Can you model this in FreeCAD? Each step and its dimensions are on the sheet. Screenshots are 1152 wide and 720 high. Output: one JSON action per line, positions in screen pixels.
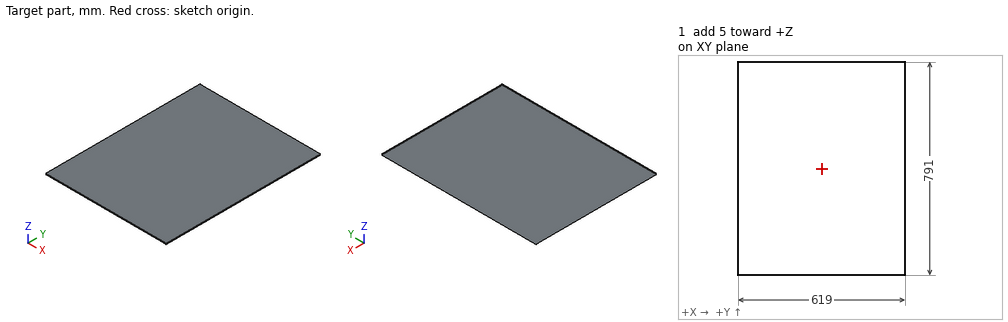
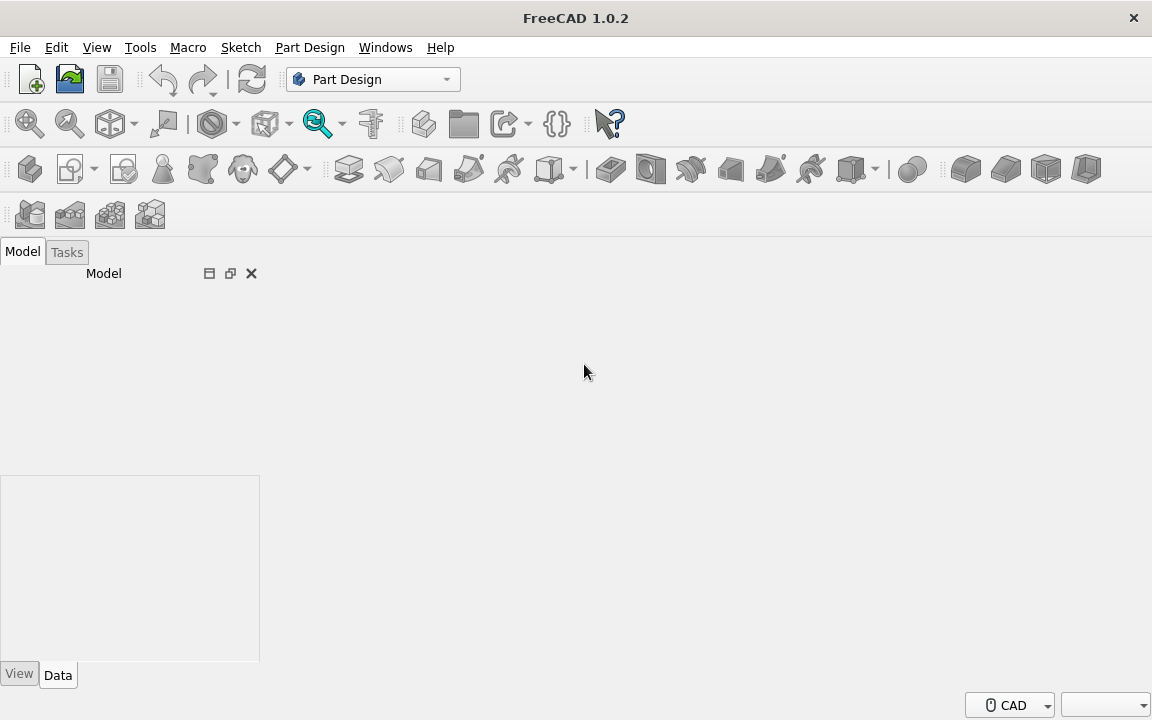
{"action": "left_click", "coordinate": [30, 80]}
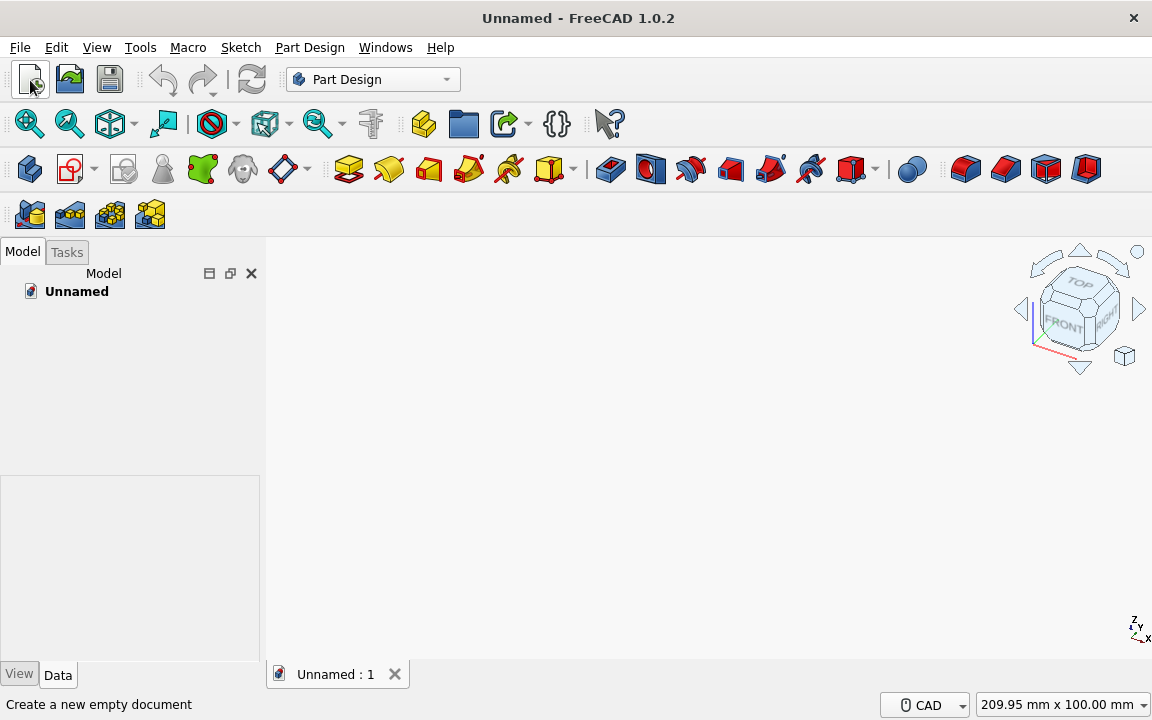
{"action": "left_click", "coordinate": [70, 170]}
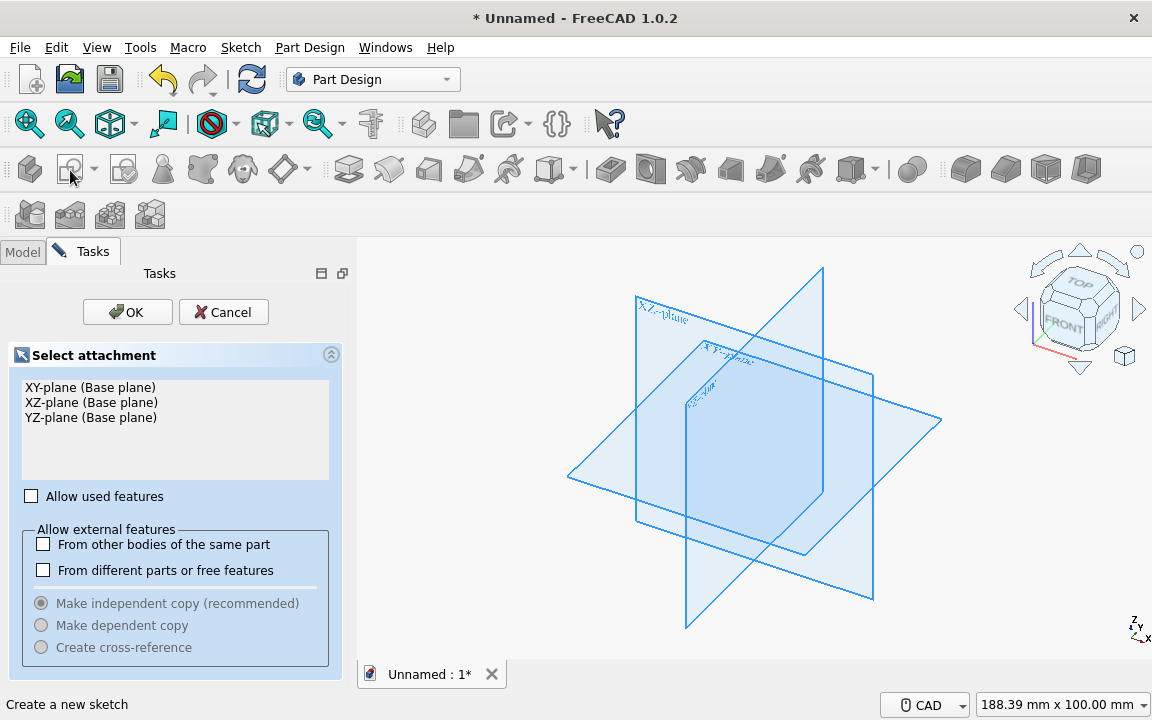
{"action": "left_click", "coordinate": [82, 388]}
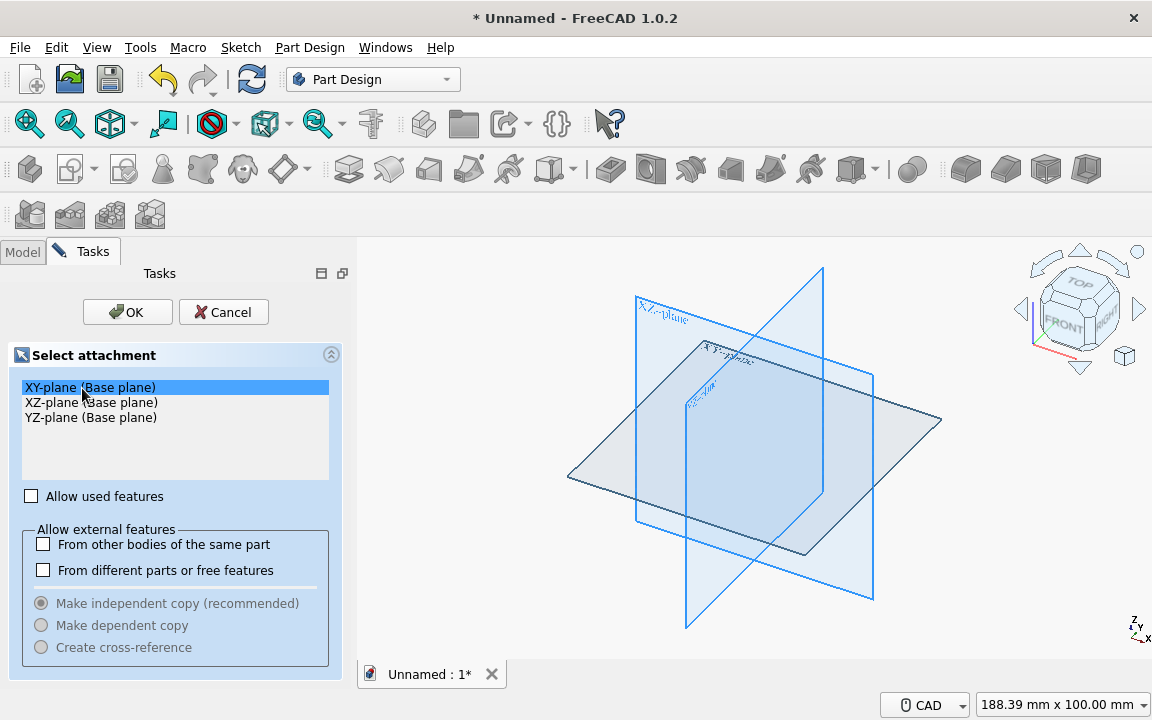
{"action": "left_click", "coordinate": [128, 312]}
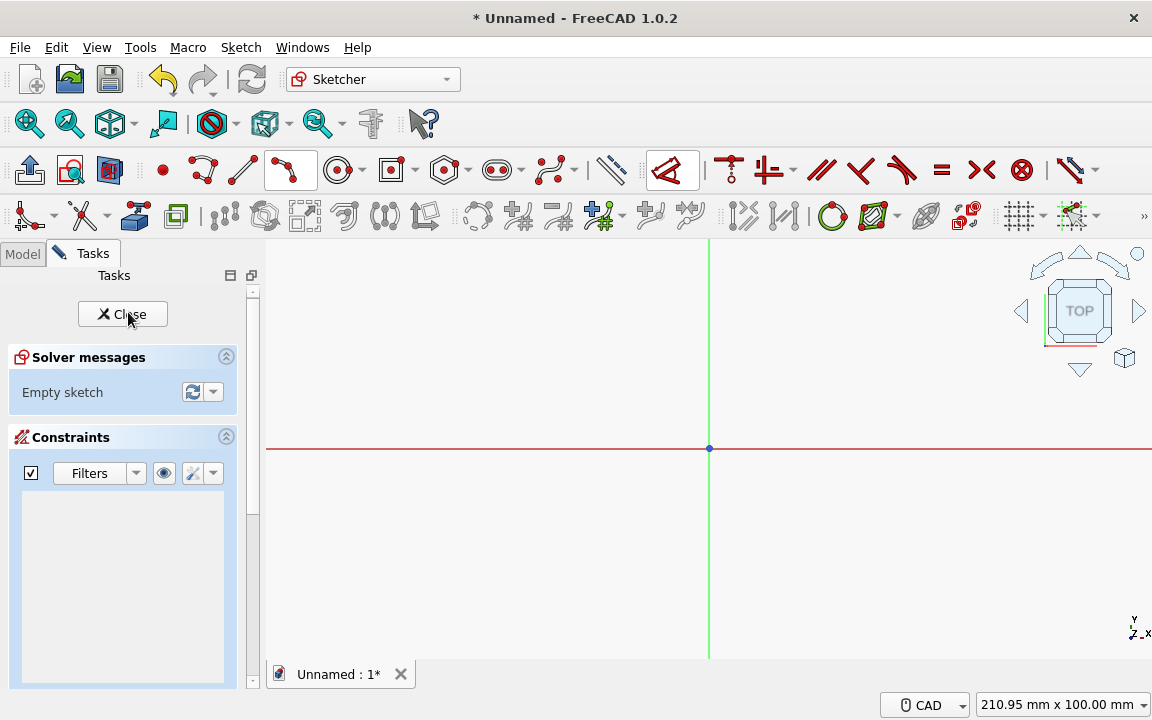
{"action": "scroll", "coordinate": [635, 449], "scroll_direction": "down", "scroll_amount": 13}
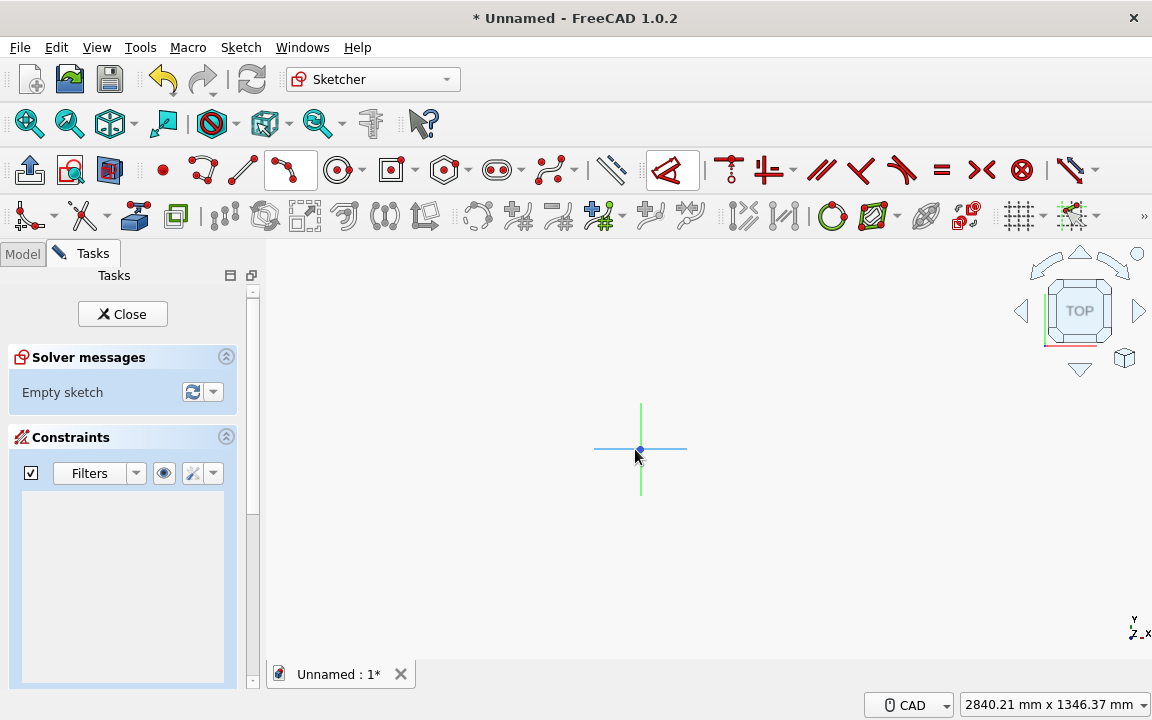
{"action": "left_click", "coordinate": [392, 170]}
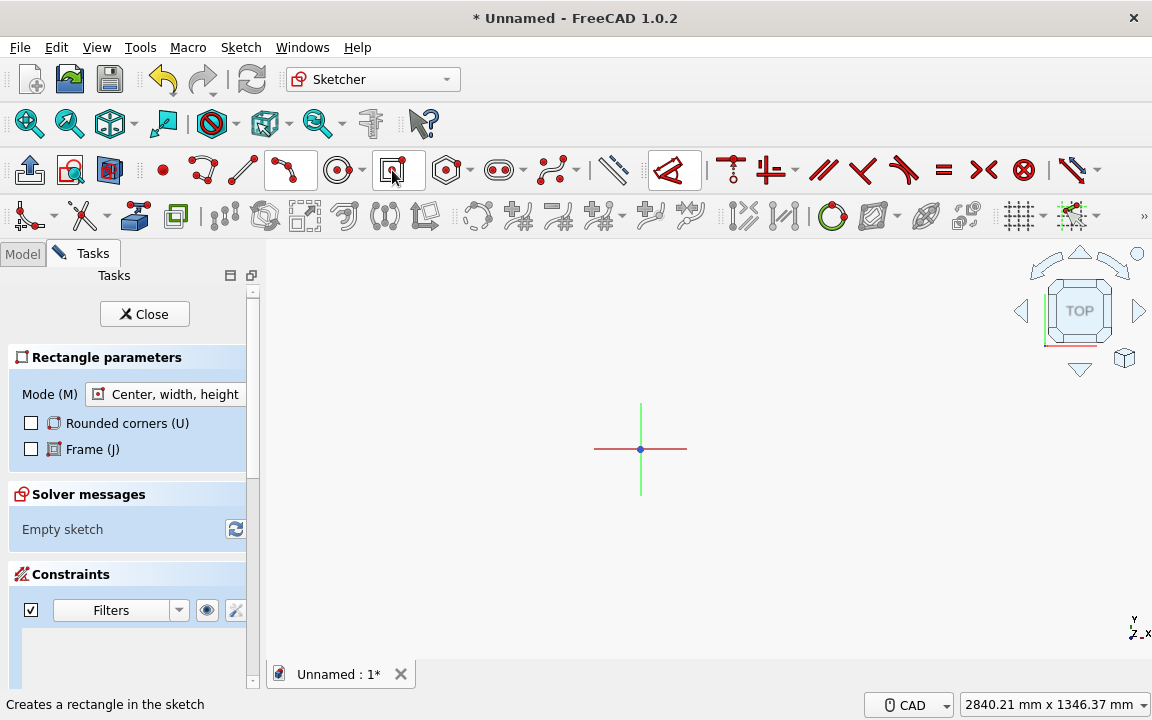
{"action": "left_click", "coordinate": [641, 449]}
{"action": "mouse_move", "coordinate": [737, 326]}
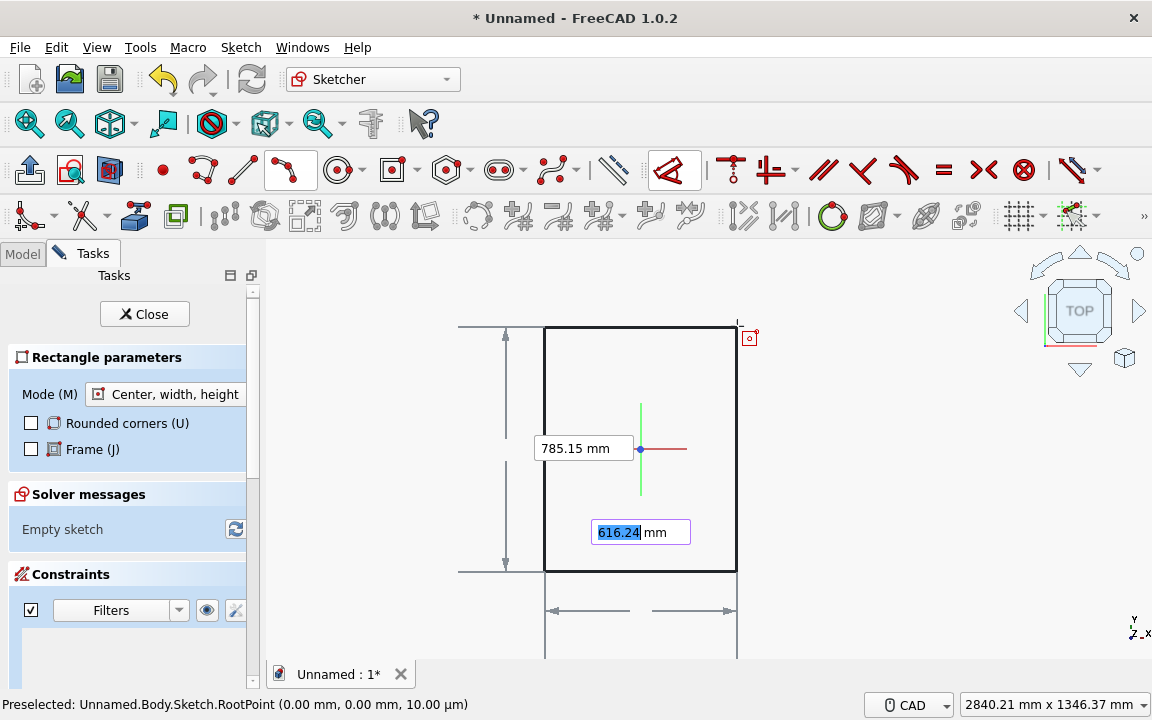
{"action": "type", "text": "619"}
{"action": "key", "text": "Tab"}
{"action": "type", "text": "791"}
{"action": "key", "text": "Return"}
{"action": "key", "text": "Escape"}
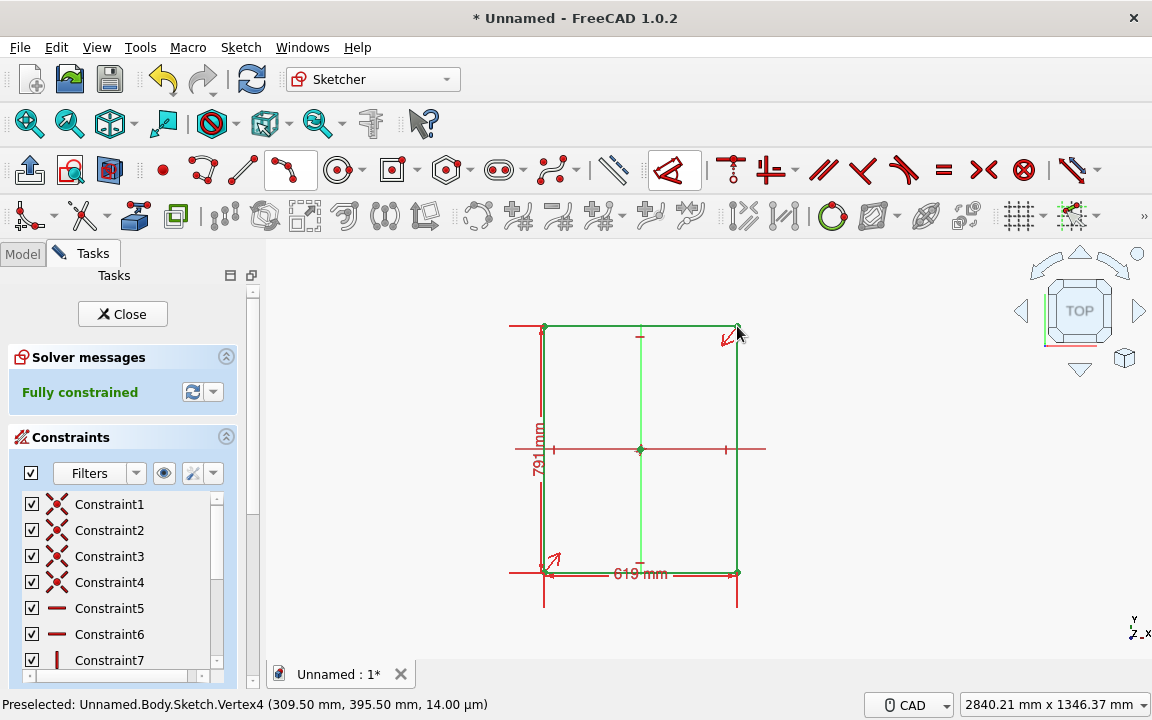
{"action": "left_click", "coordinate": [123, 314]}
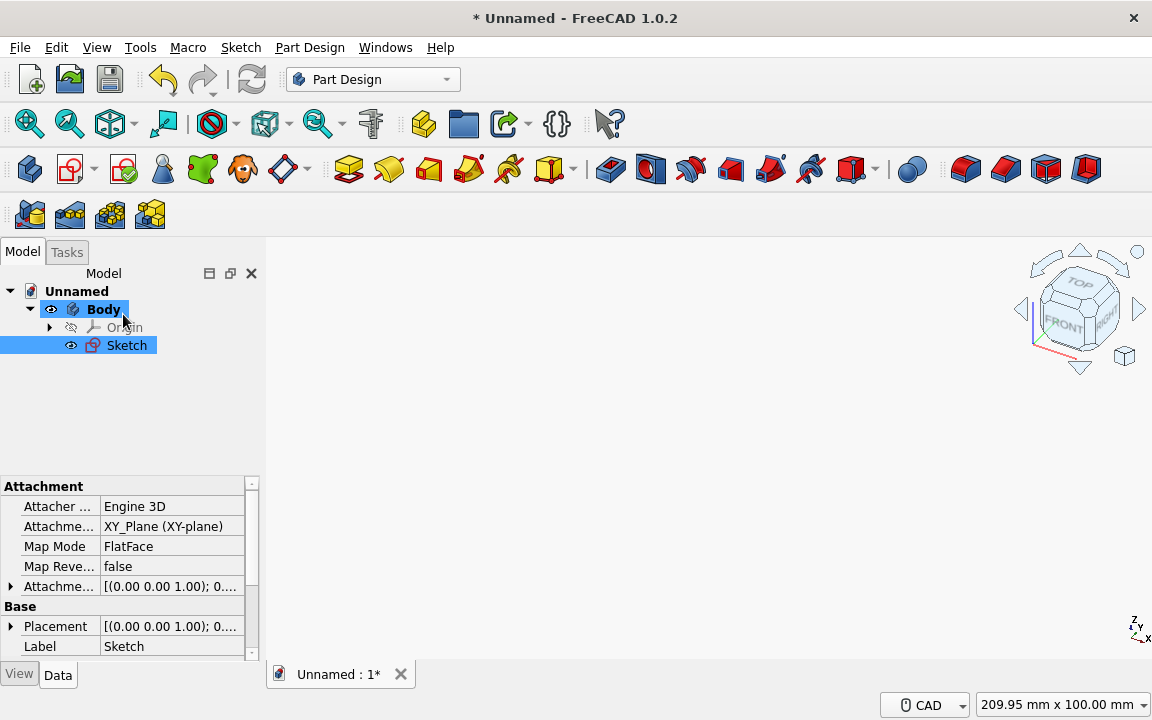
{"action": "left_click", "coordinate": [350, 170]}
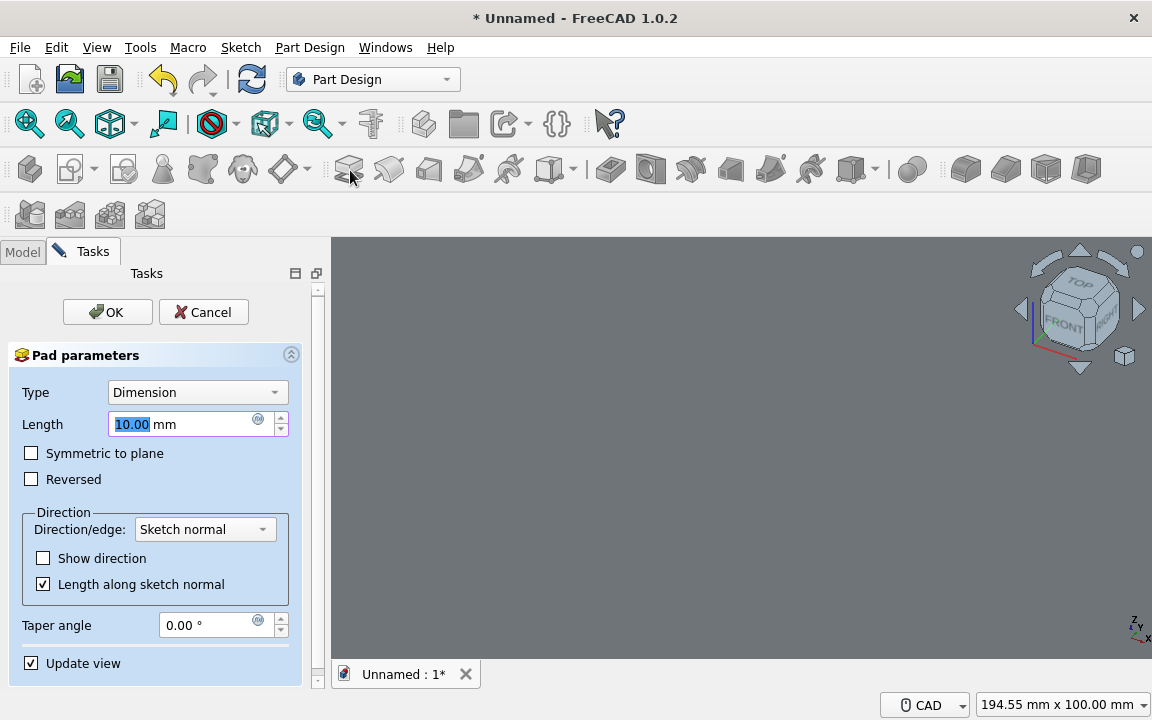
{"action": "type", "text": "5"}
{"action": "key", "text": "Tab"}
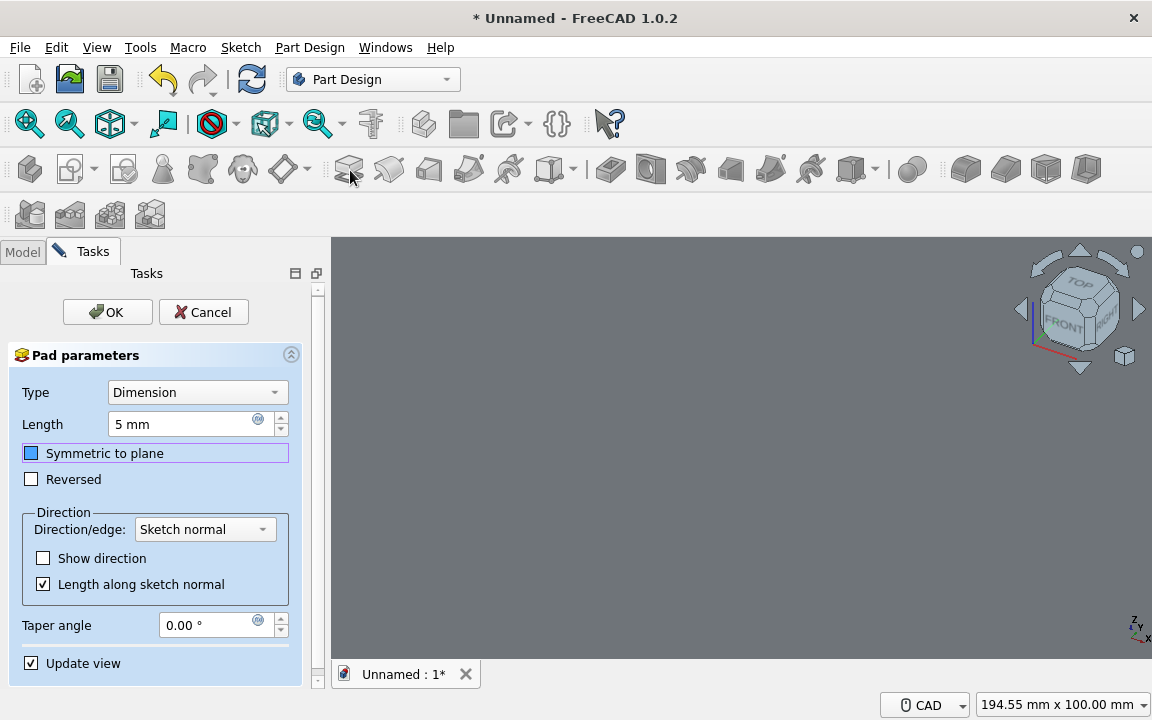
{"action": "left_click", "coordinate": [108, 312]}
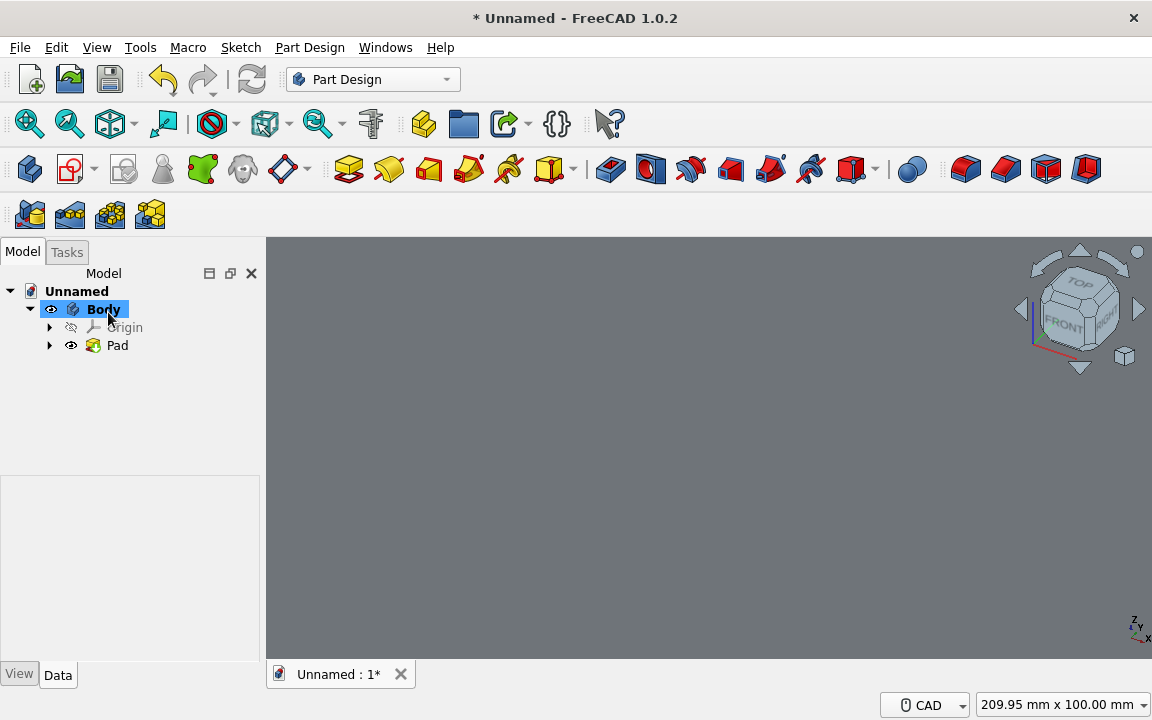
{"action": "key", "text": "0"}